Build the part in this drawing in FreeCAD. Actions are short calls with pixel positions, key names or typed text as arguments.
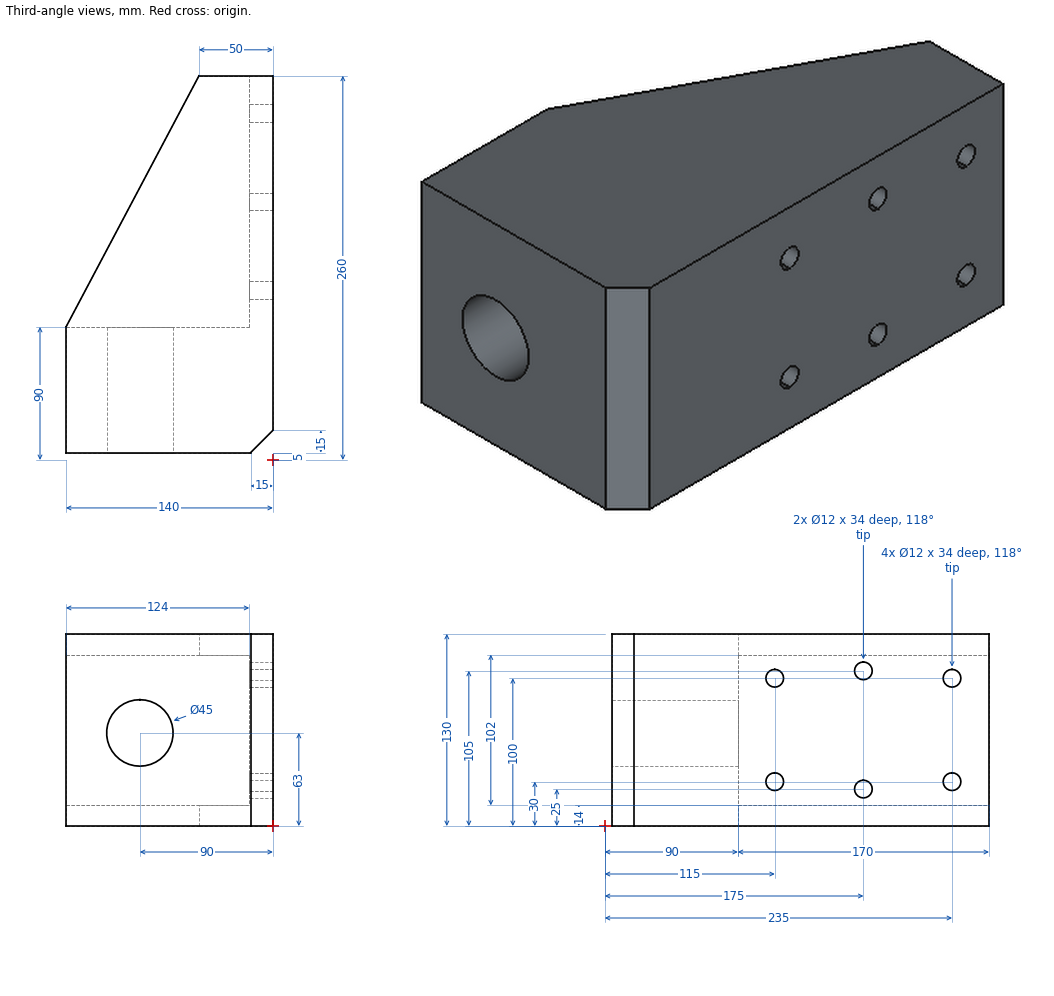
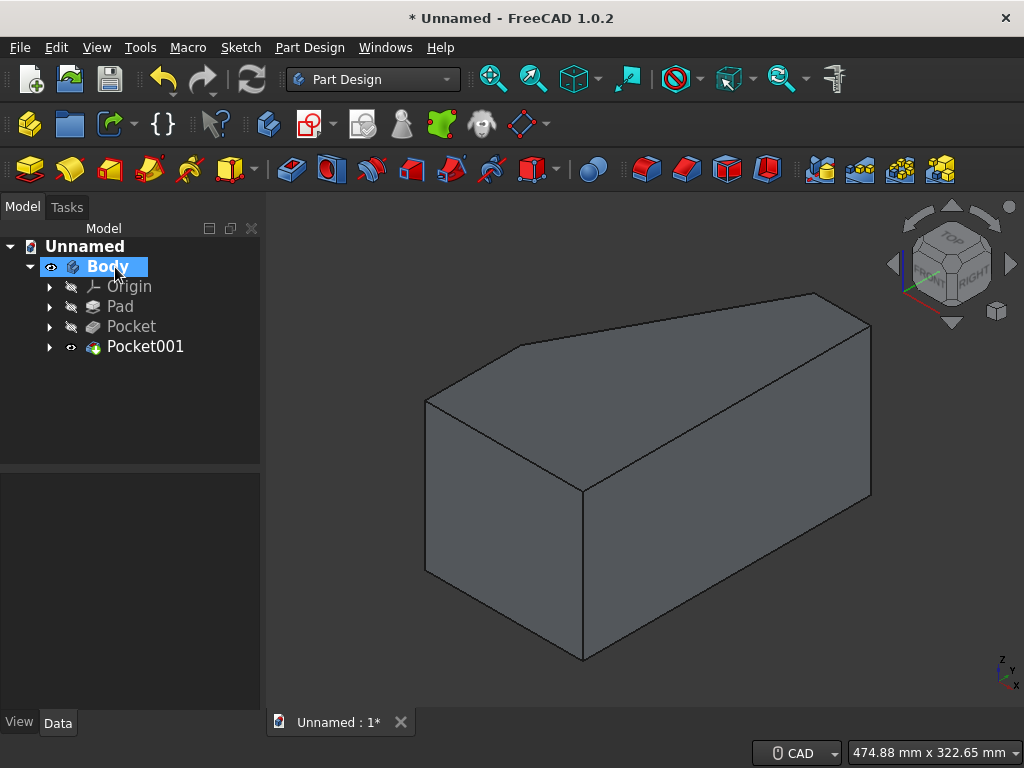
click(607, 386)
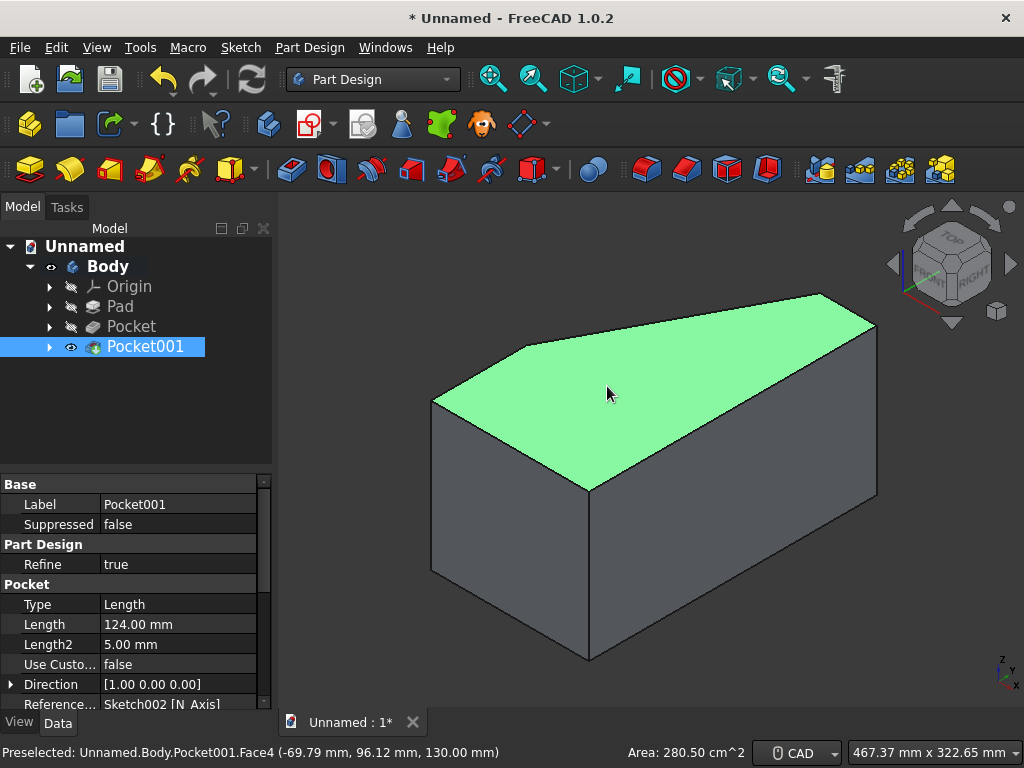
click(310, 124)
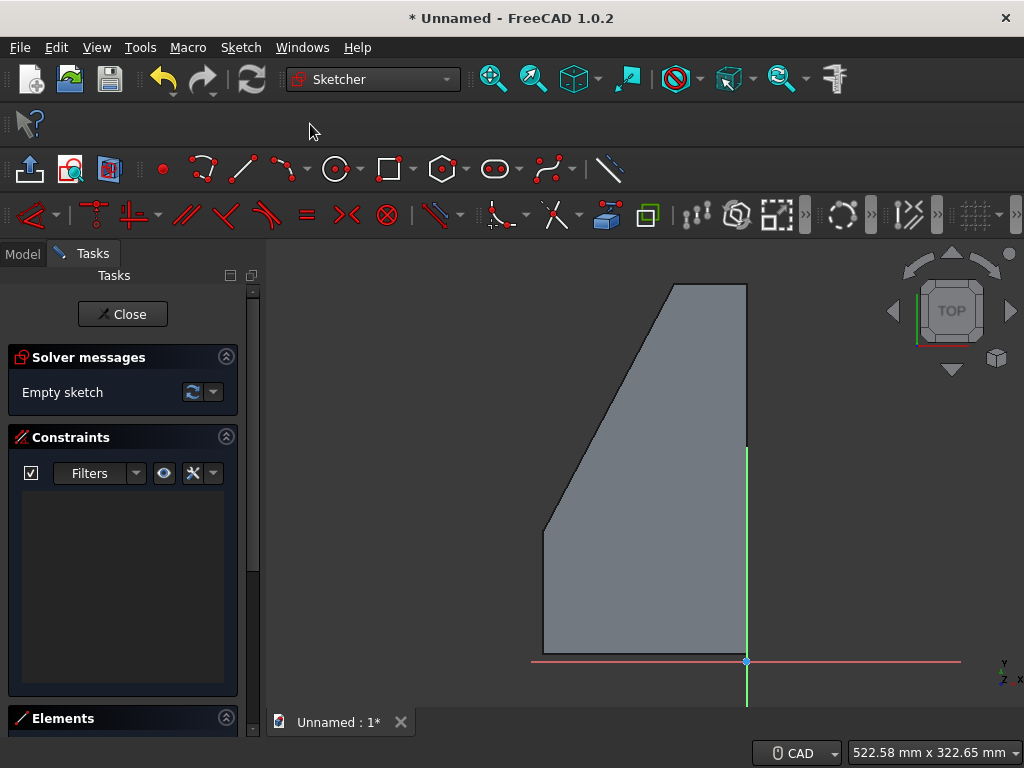
scroll(752, 664, up, 12)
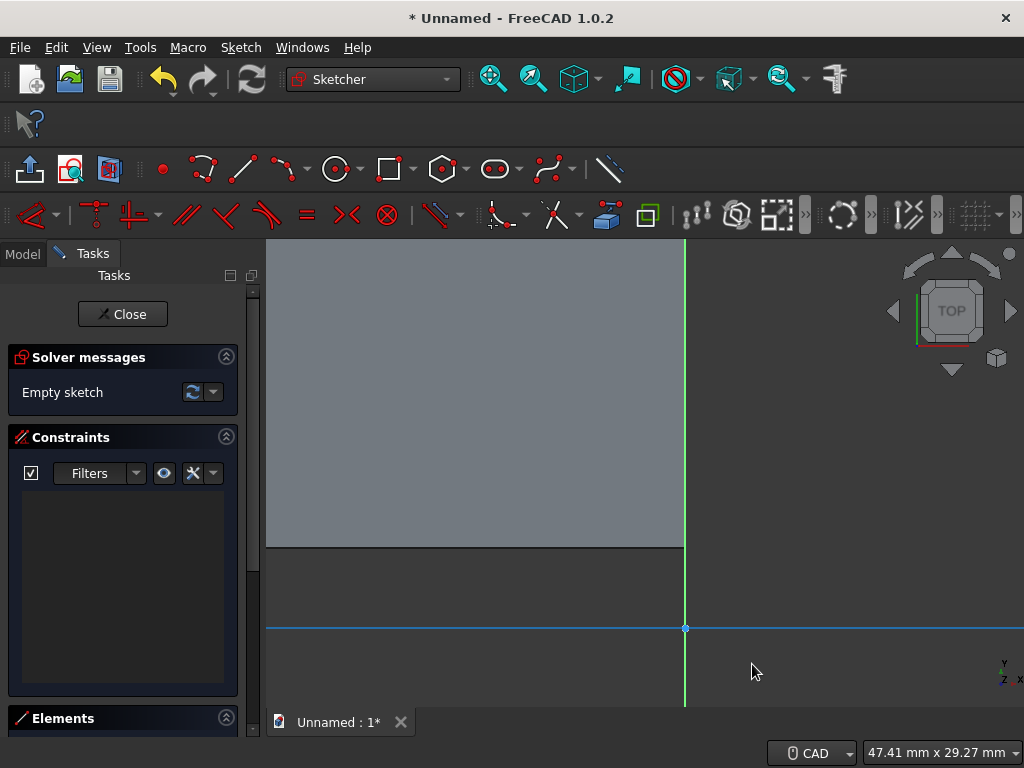
click(204, 170)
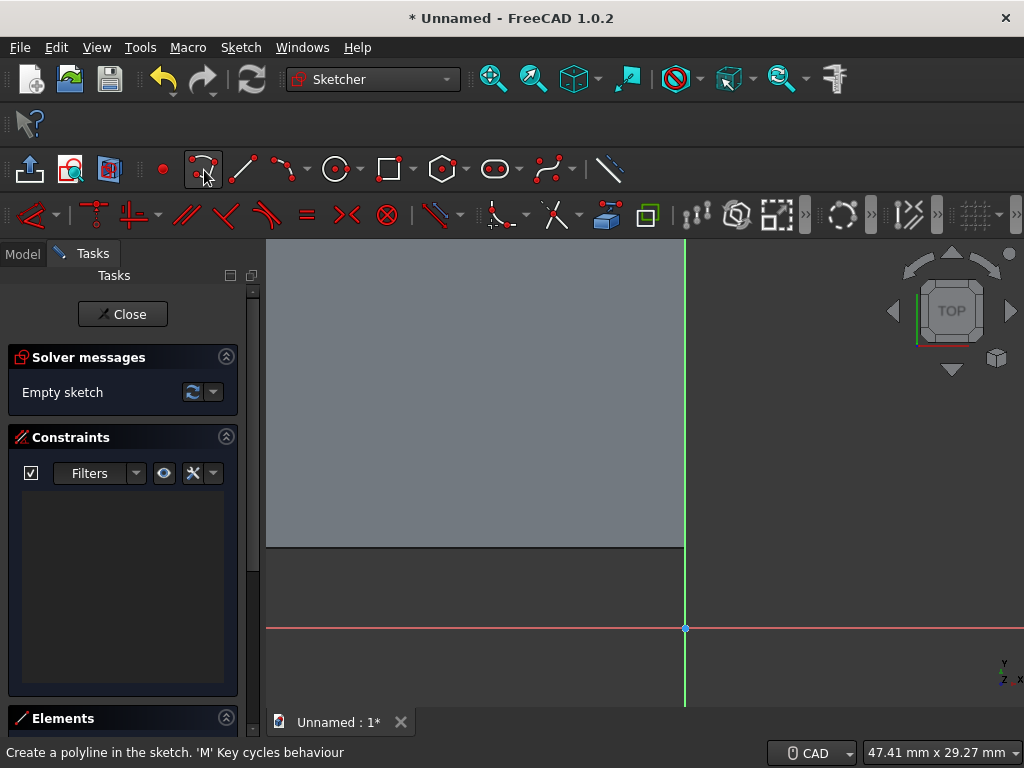
click(685, 548)
click(676, 308)
click(445, 548)
click(685, 549)
key(Escape)
key(Escape)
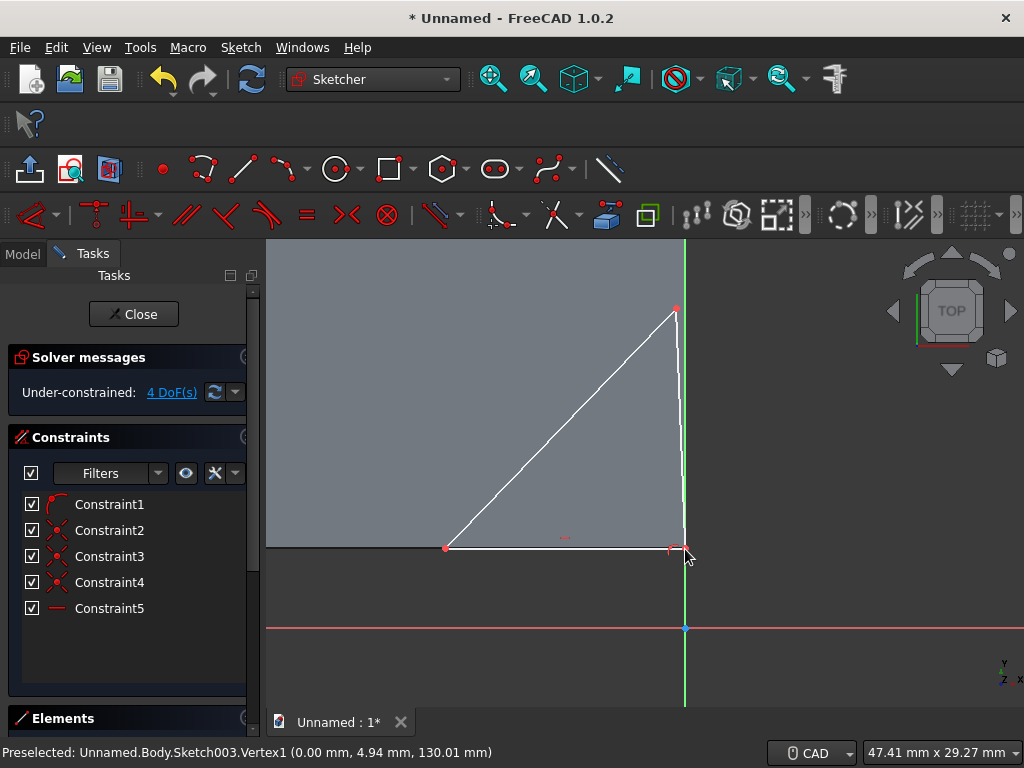
click(683, 477)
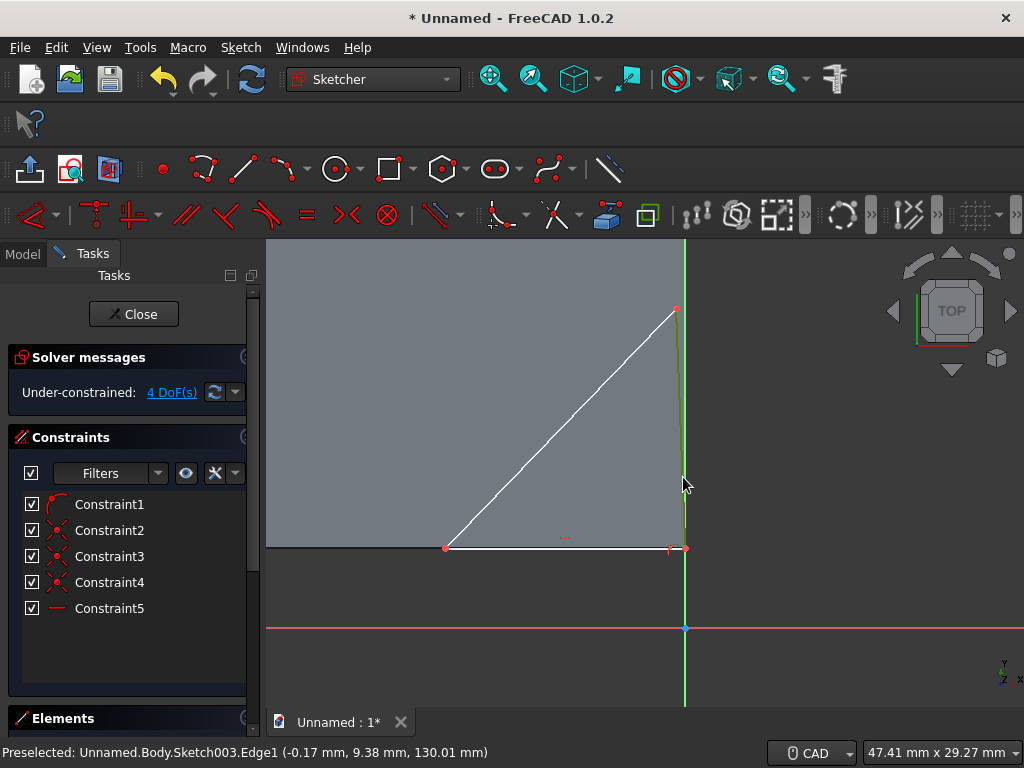
click(160, 216)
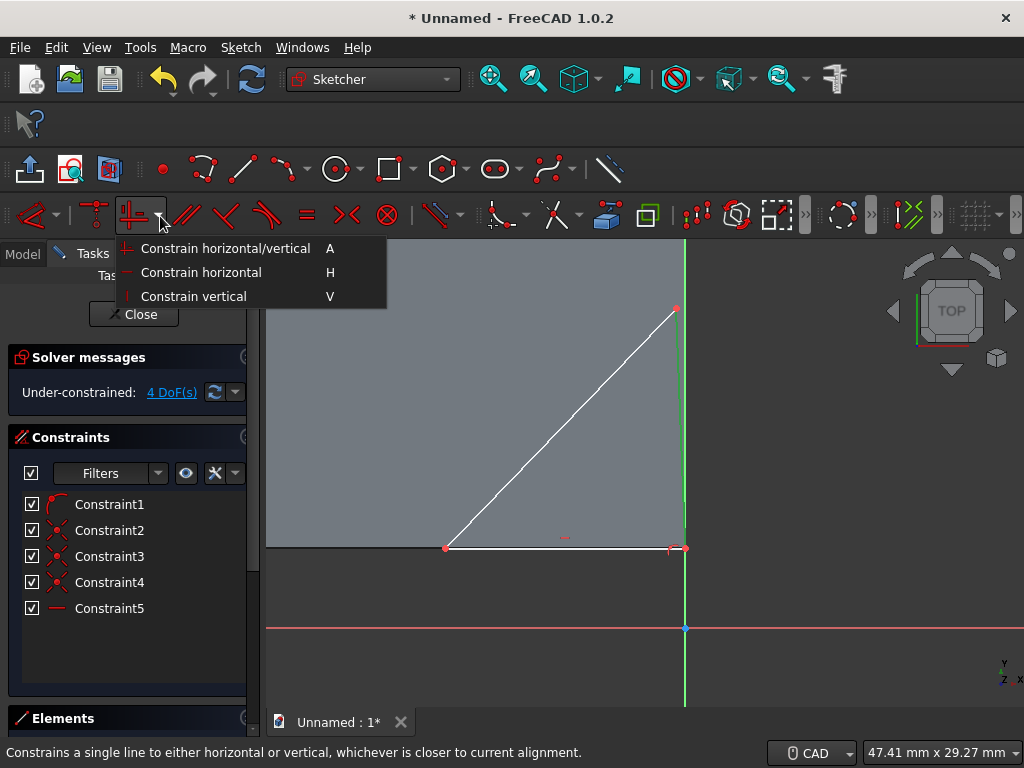
click(251, 296)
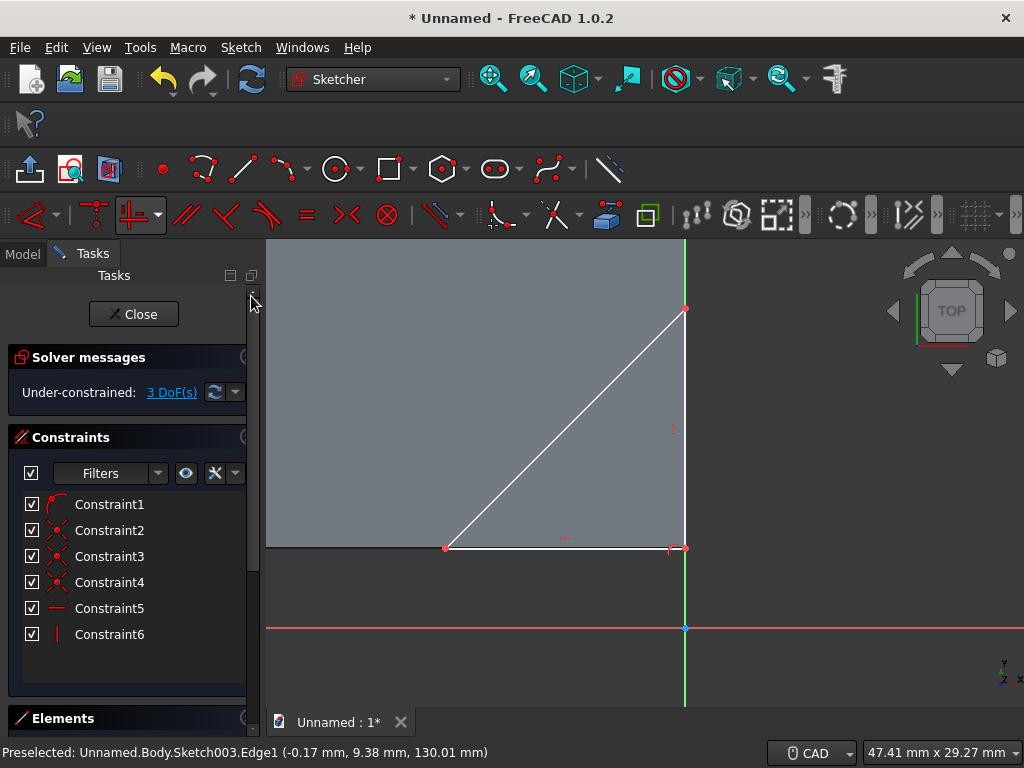
click(32, 216)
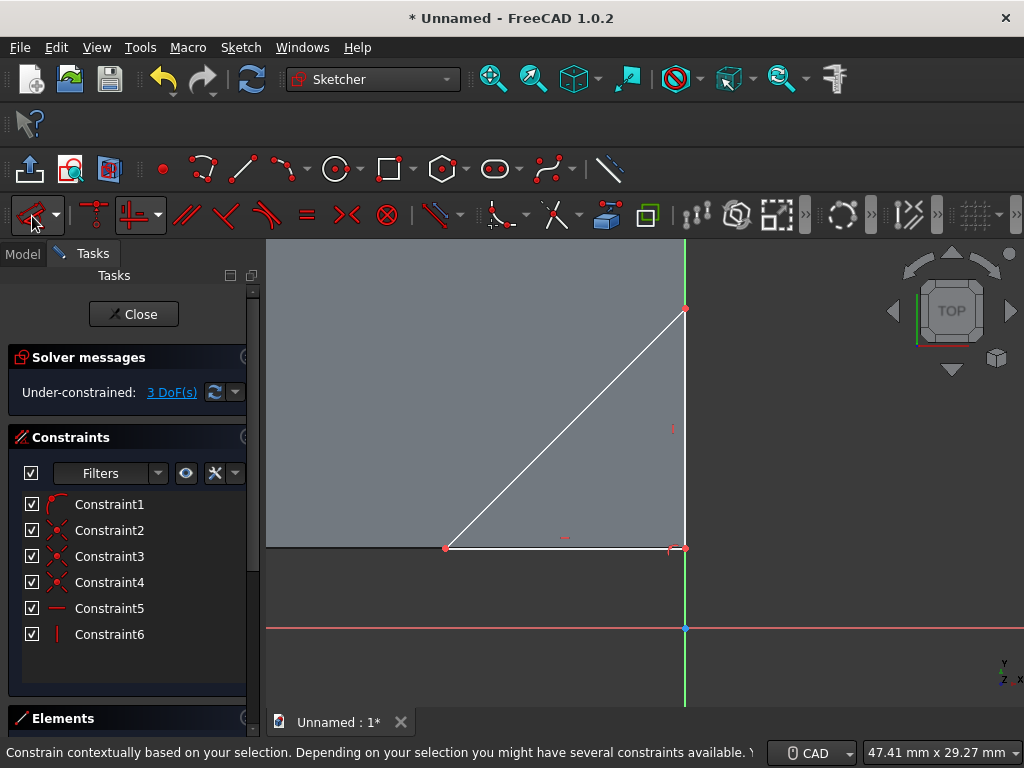
click(685, 477)
click(719, 429)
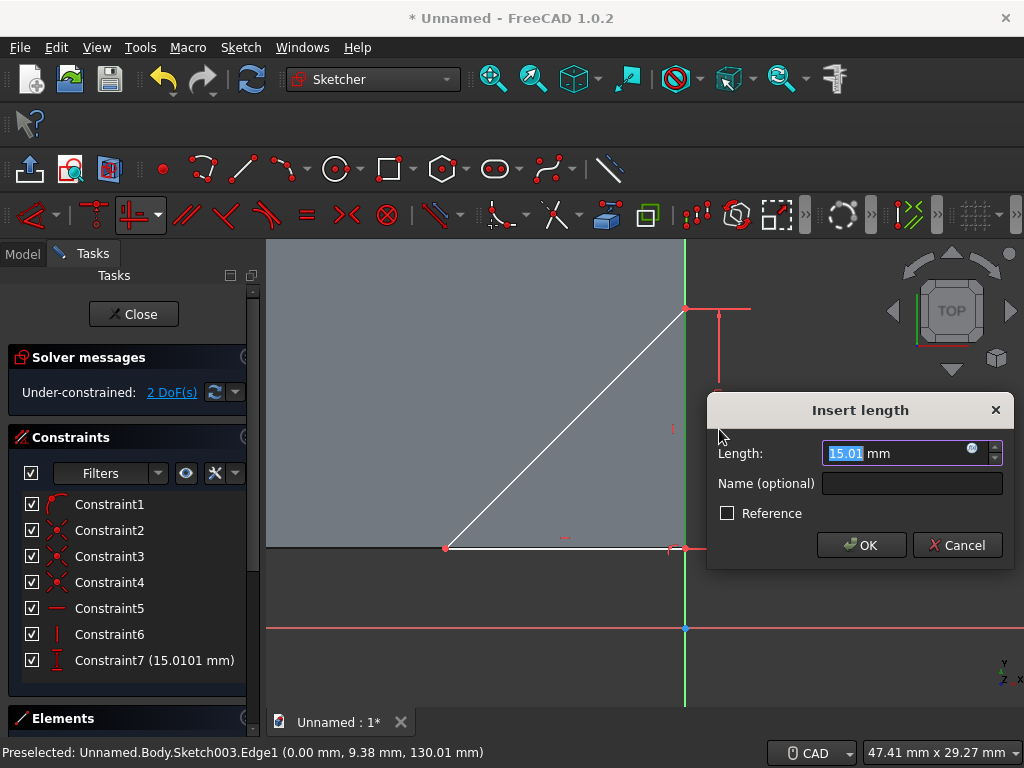
text(15)
key(Return)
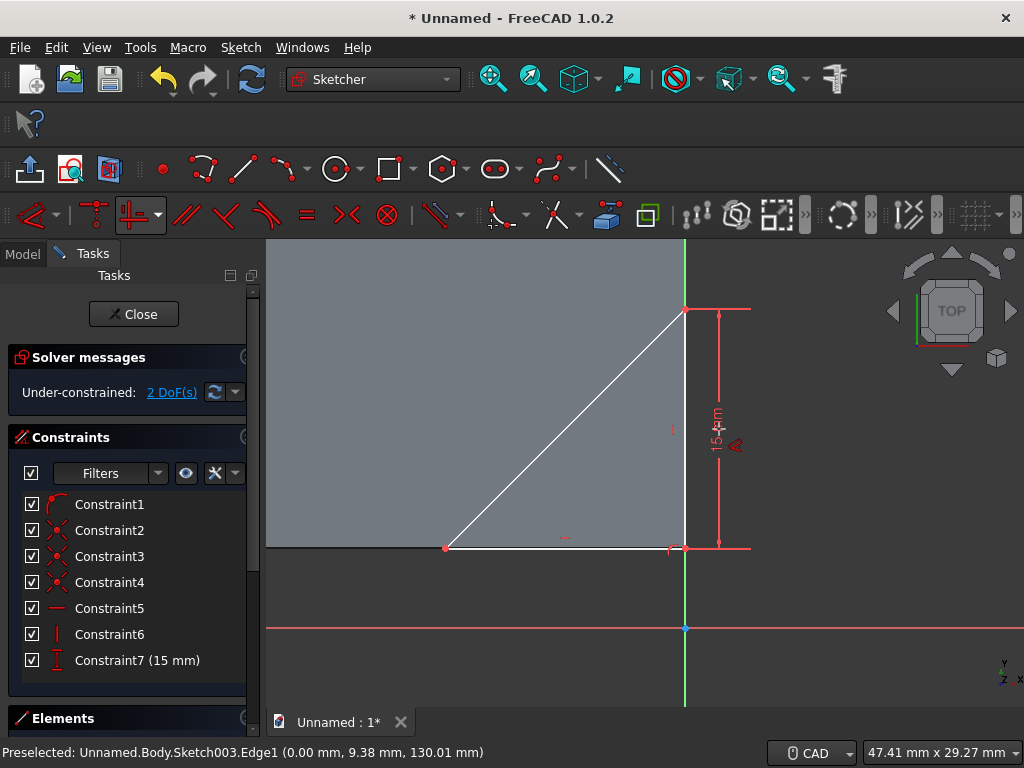
click(517, 549)
click(565, 583)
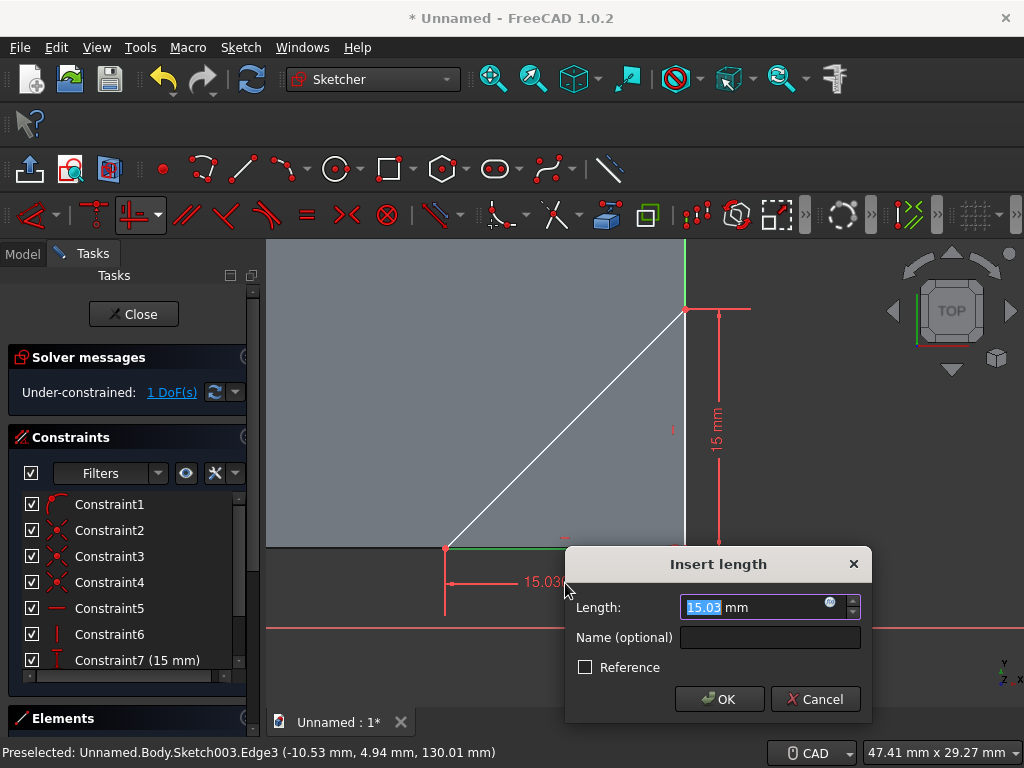
text(15)
key(Return)